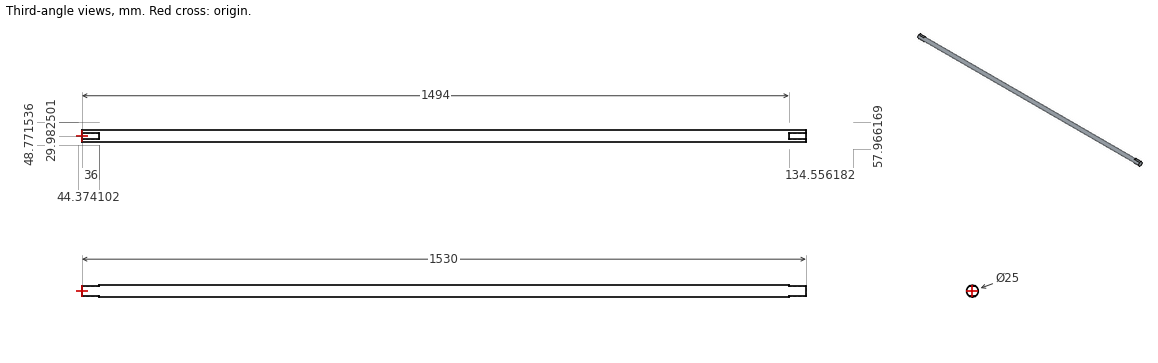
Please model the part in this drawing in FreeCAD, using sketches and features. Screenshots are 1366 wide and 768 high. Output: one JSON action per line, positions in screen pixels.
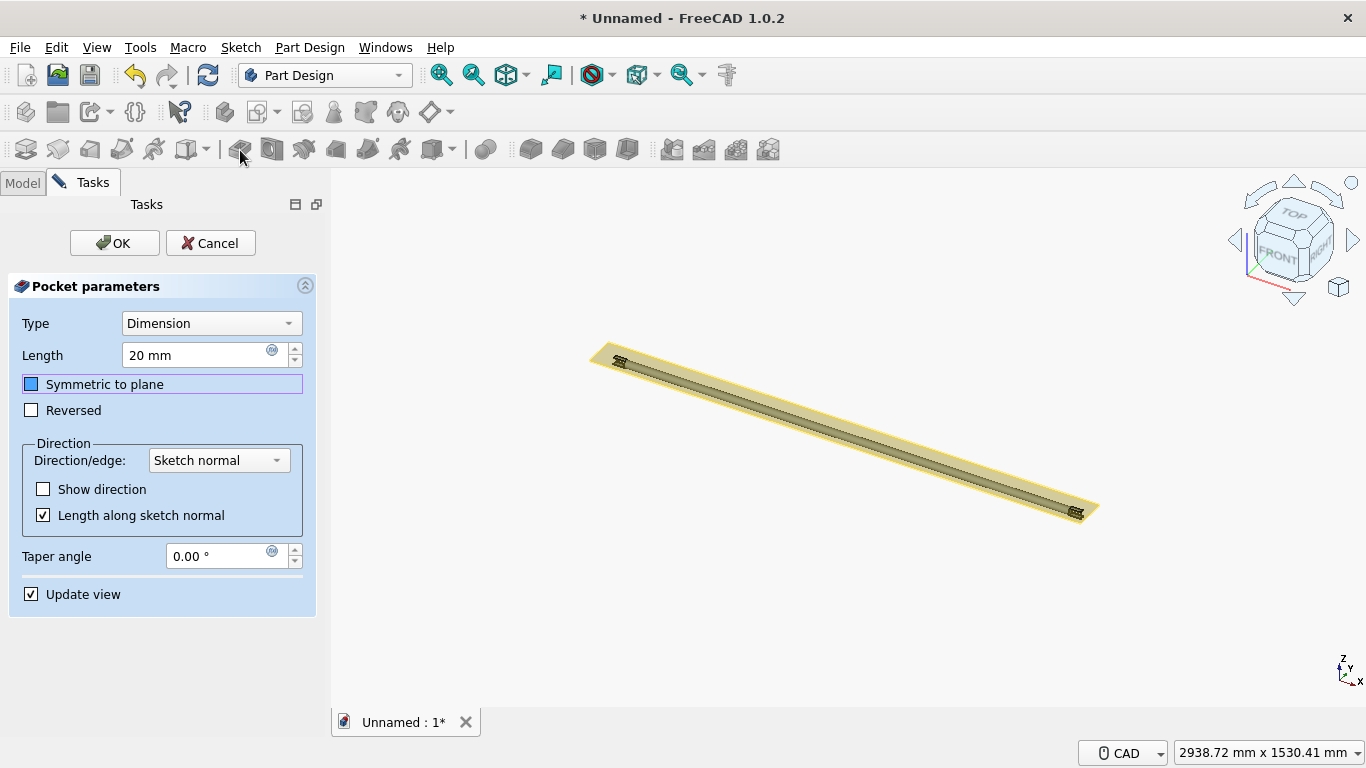
{"action": "left_click", "coordinate": [30, 410]}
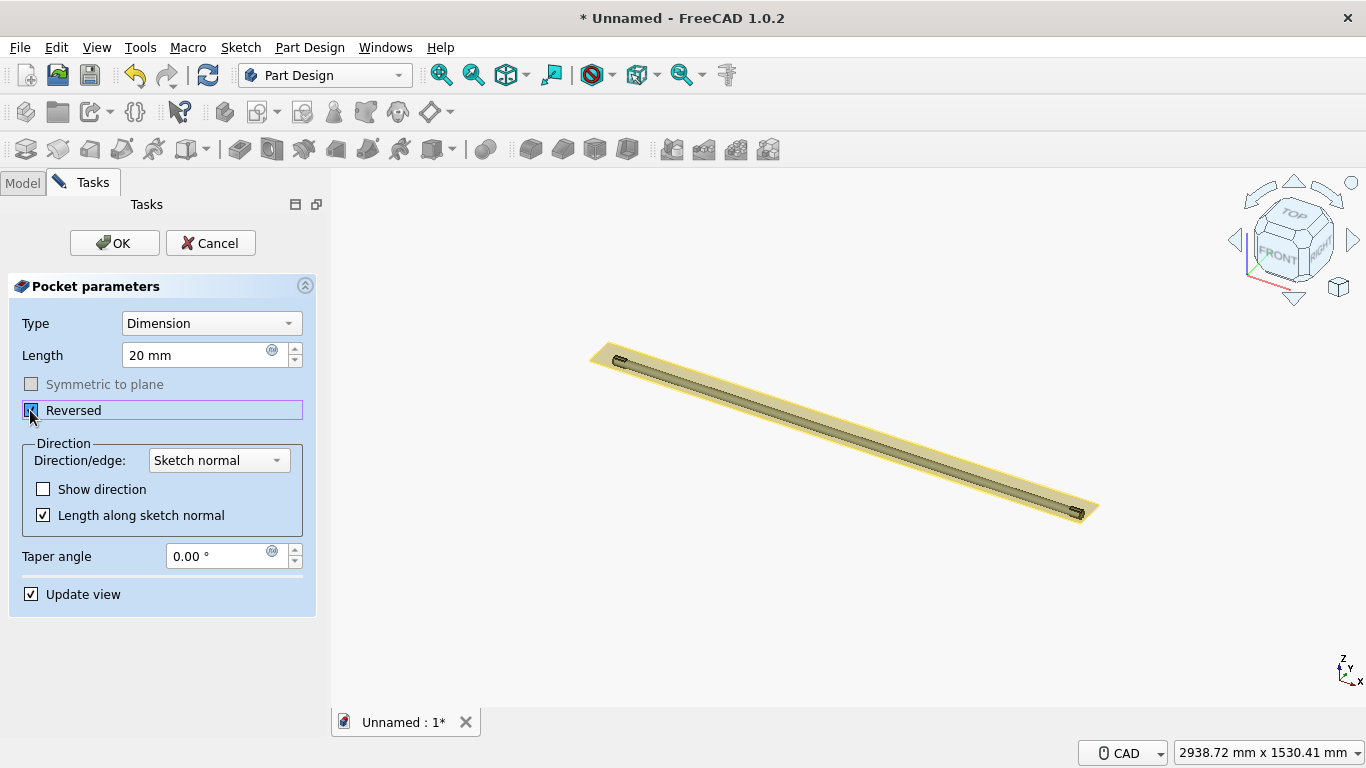
{"action": "left_click", "coordinate": [115, 243]}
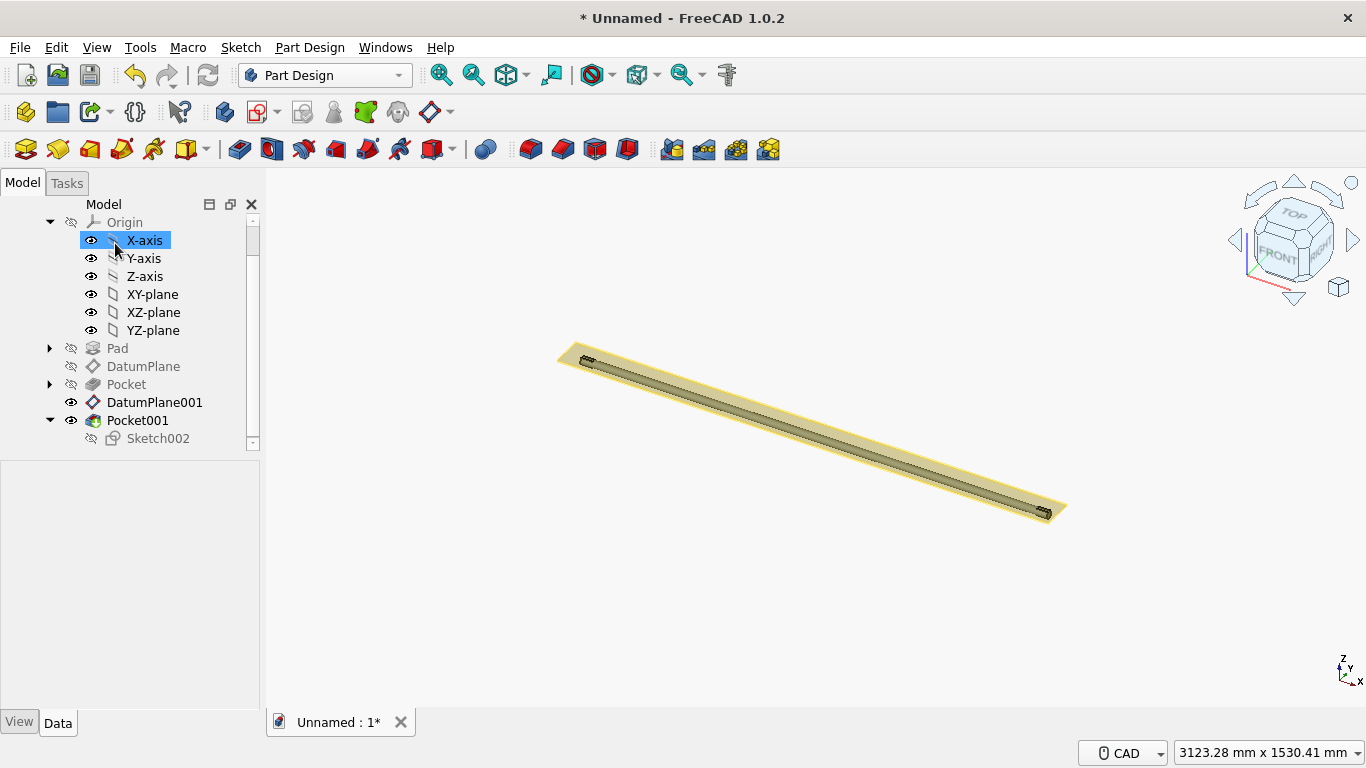
{"action": "left_click", "coordinate": [116, 402]}
{"action": "key", "text": "space"}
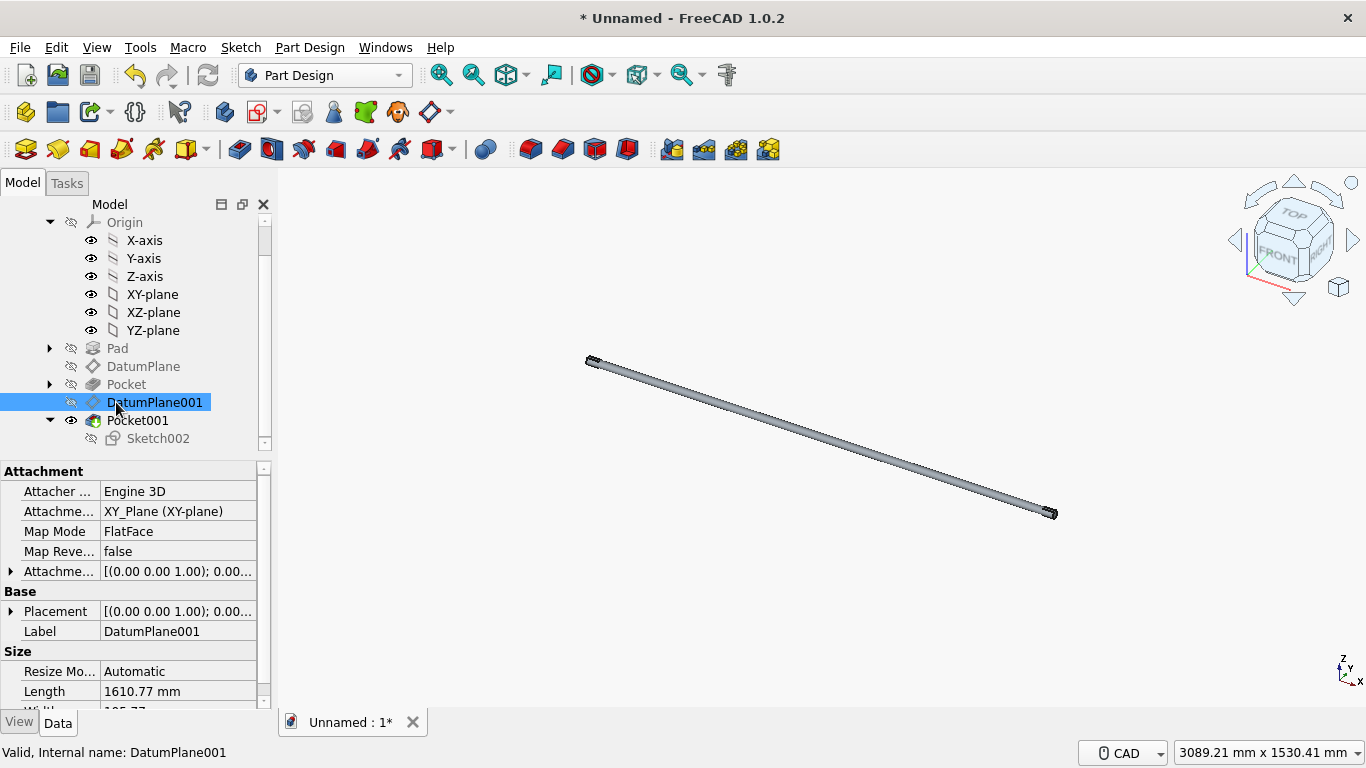
{"action": "key", "text": "0"}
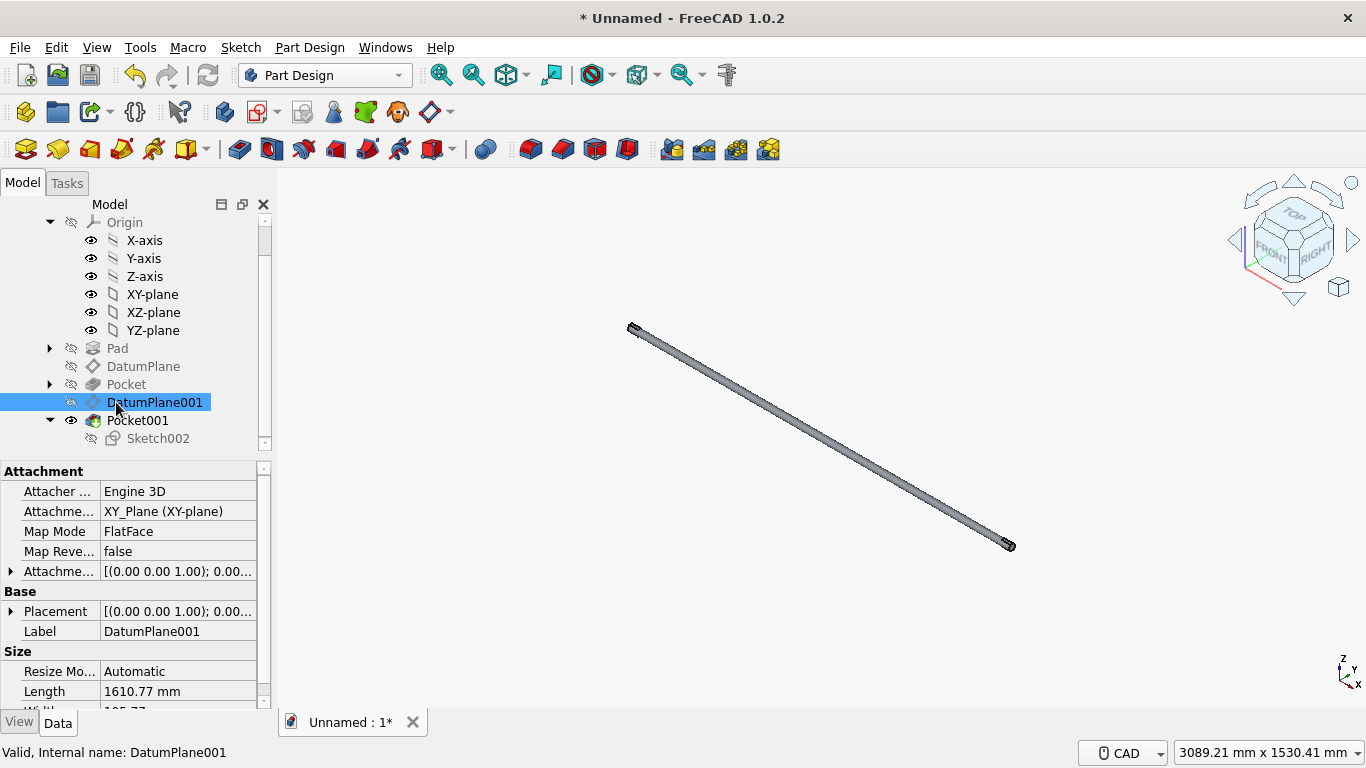
{"action": "left_click", "coordinate": [442, 76]}